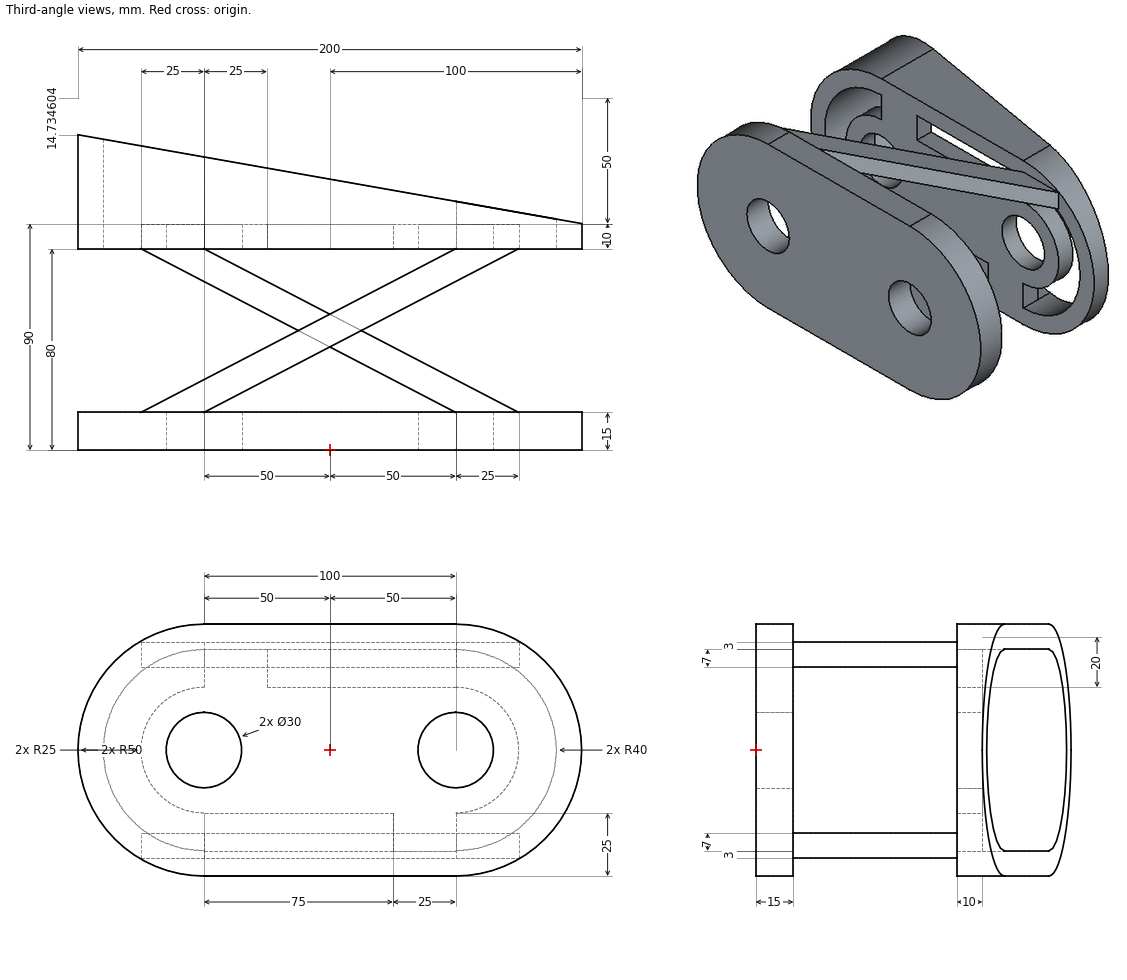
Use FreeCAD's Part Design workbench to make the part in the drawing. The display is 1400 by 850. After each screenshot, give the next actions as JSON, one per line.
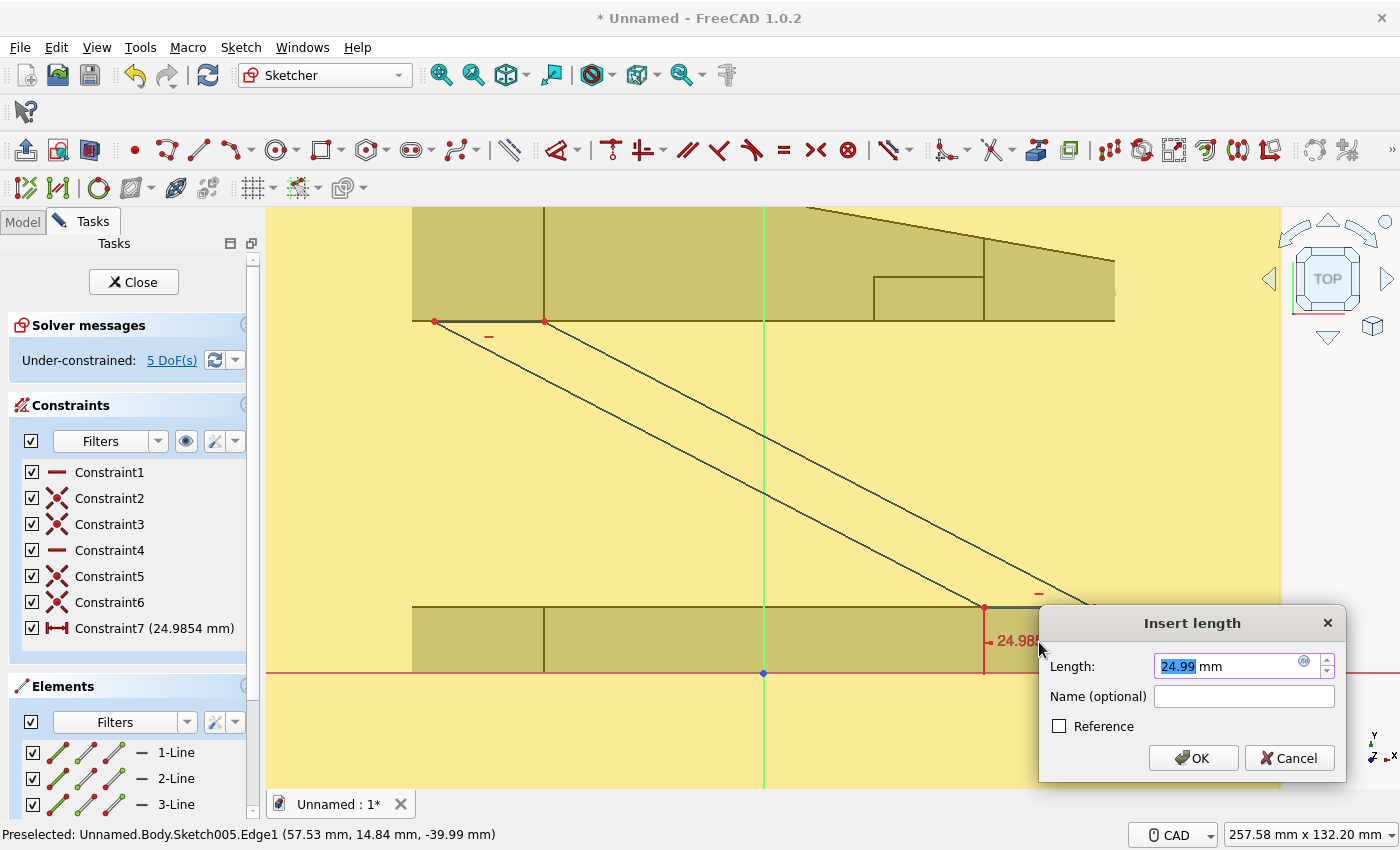
{"action": "type", "text": "25"}
{"action": "key", "text": "Return"}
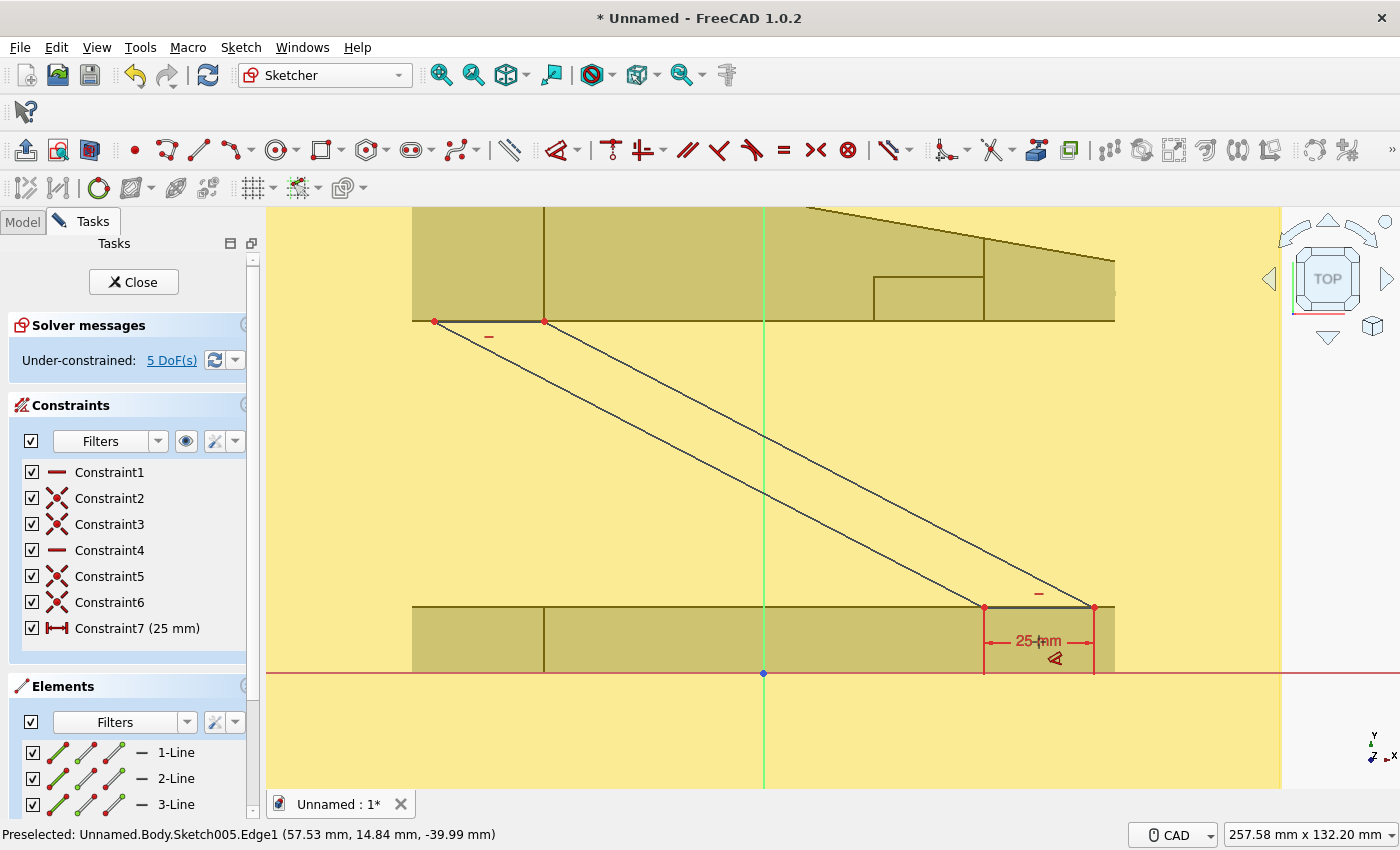
{"action": "left_click", "coordinate": [511, 322]}
{"action": "left_click", "coordinate": [489, 288]}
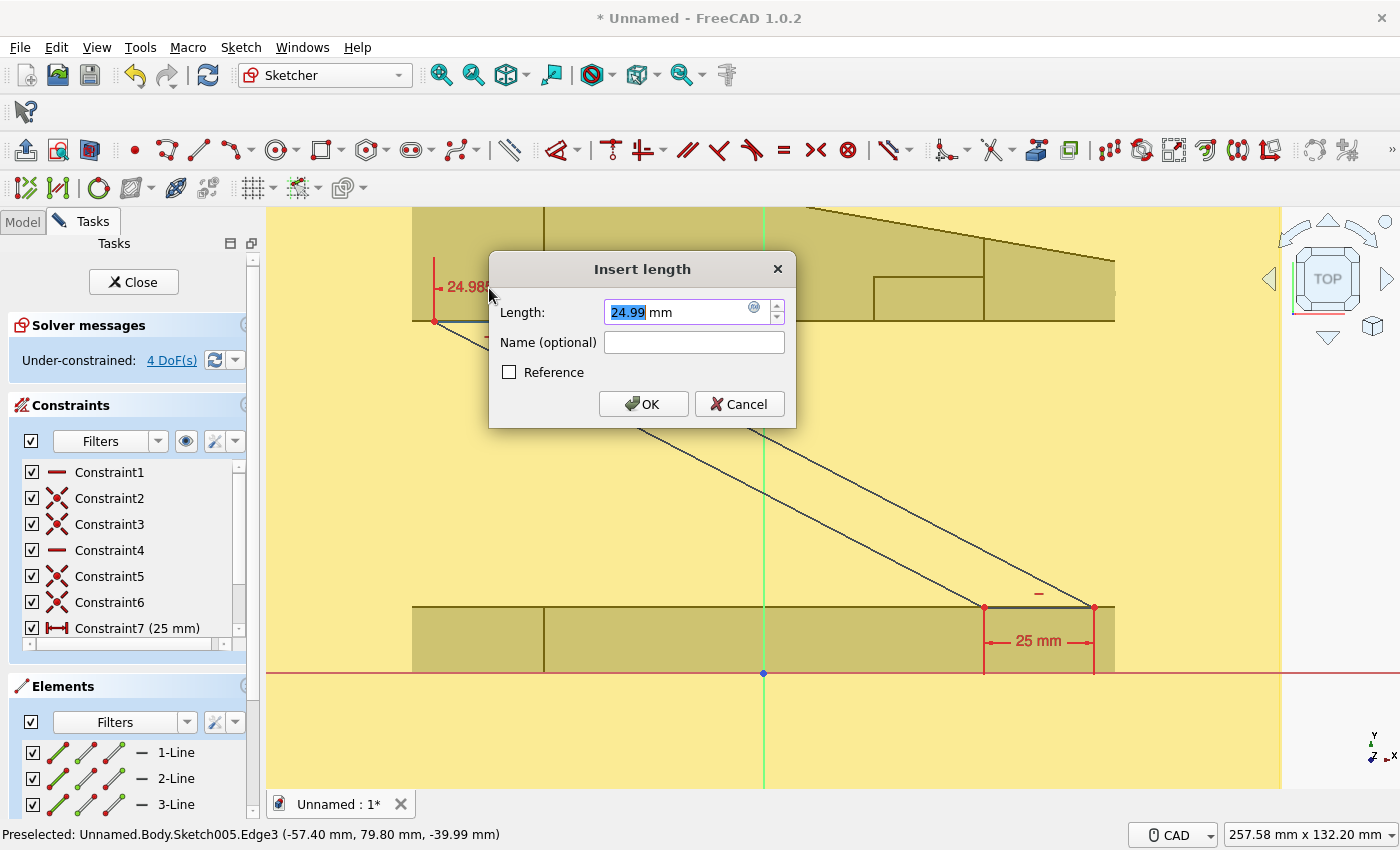
{"action": "type", "text": "25"}
{"action": "key", "text": "Return"}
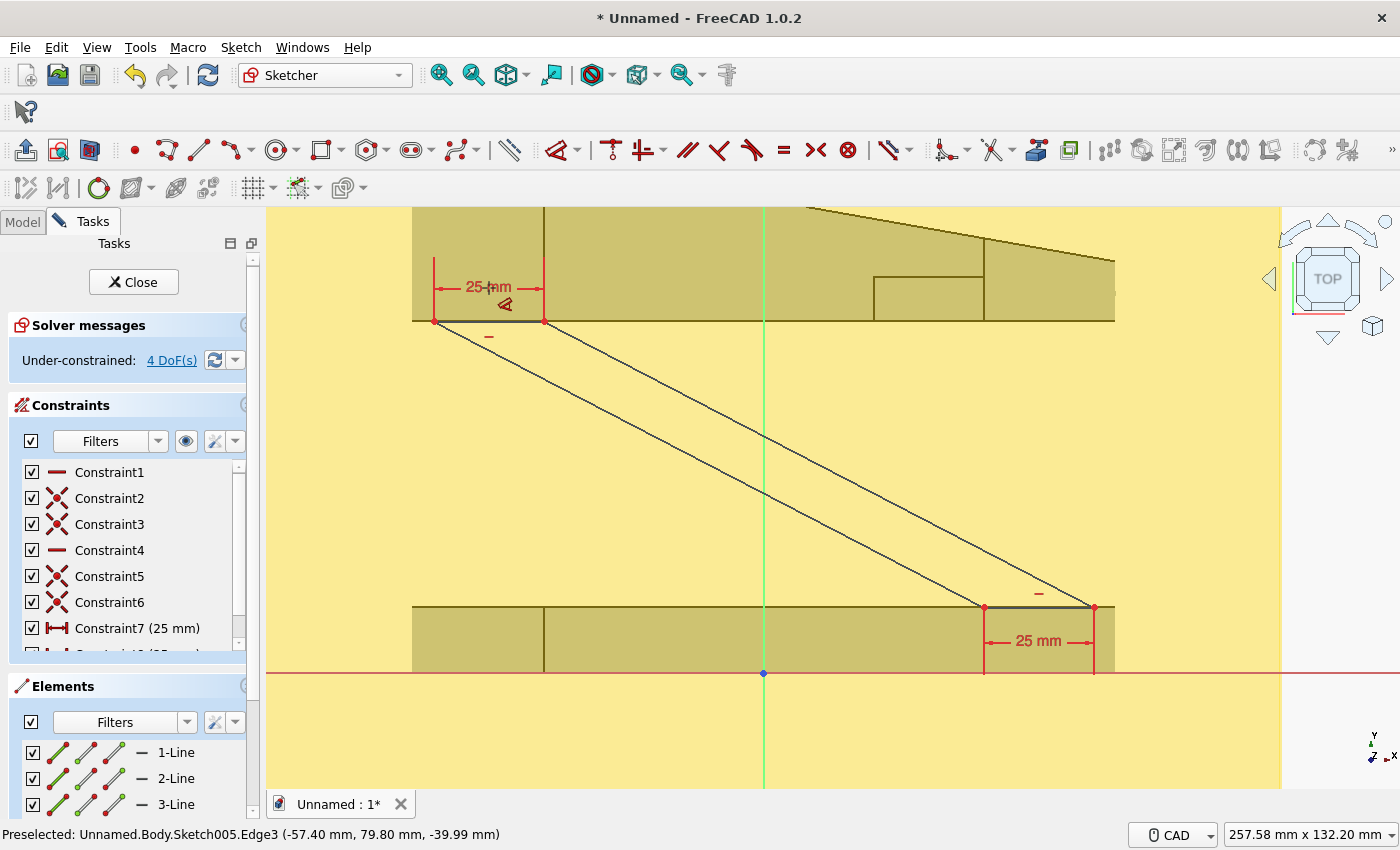
{"action": "left_click", "coordinate": [984, 608]}
{"action": "left_click", "coordinate": [874, 707]}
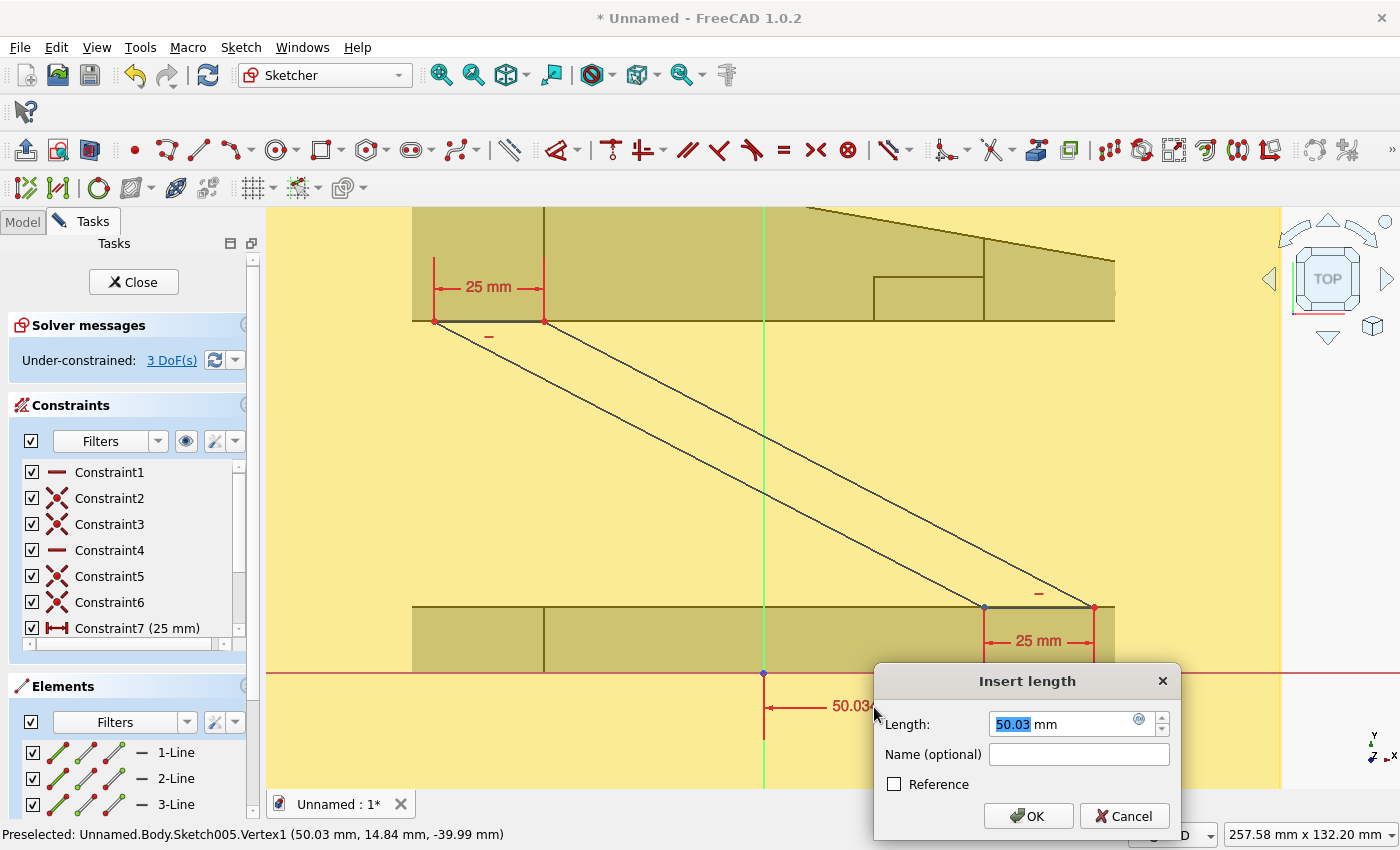
{"action": "type", "text": "50"}
{"action": "key", "text": "Return"}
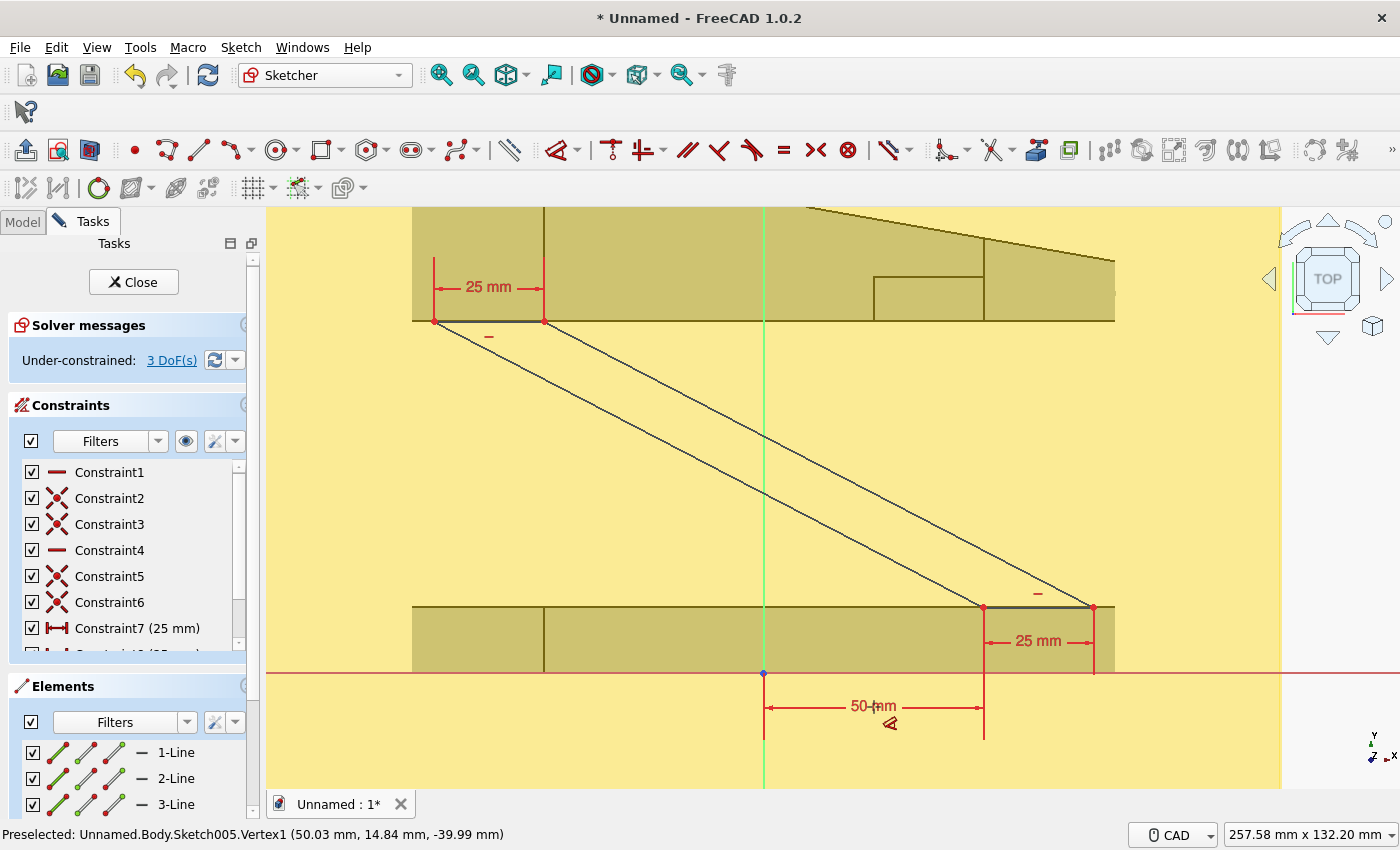
{"action": "left_click", "coordinate": [984, 608]}
{"action": "left_click", "coordinate": [730, 641]}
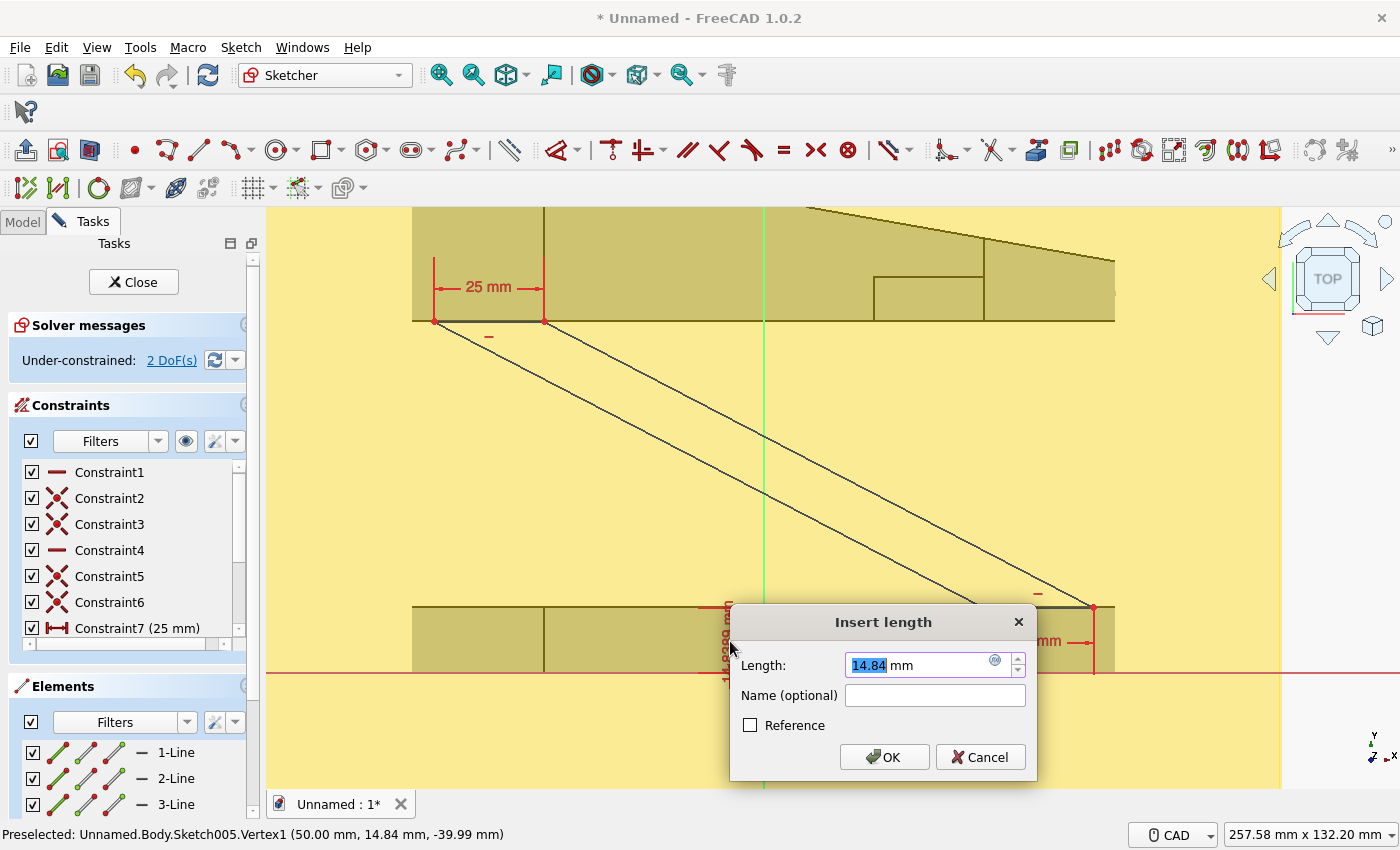
{"action": "type", "text": "15"}
{"action": "key", "text": "Return"}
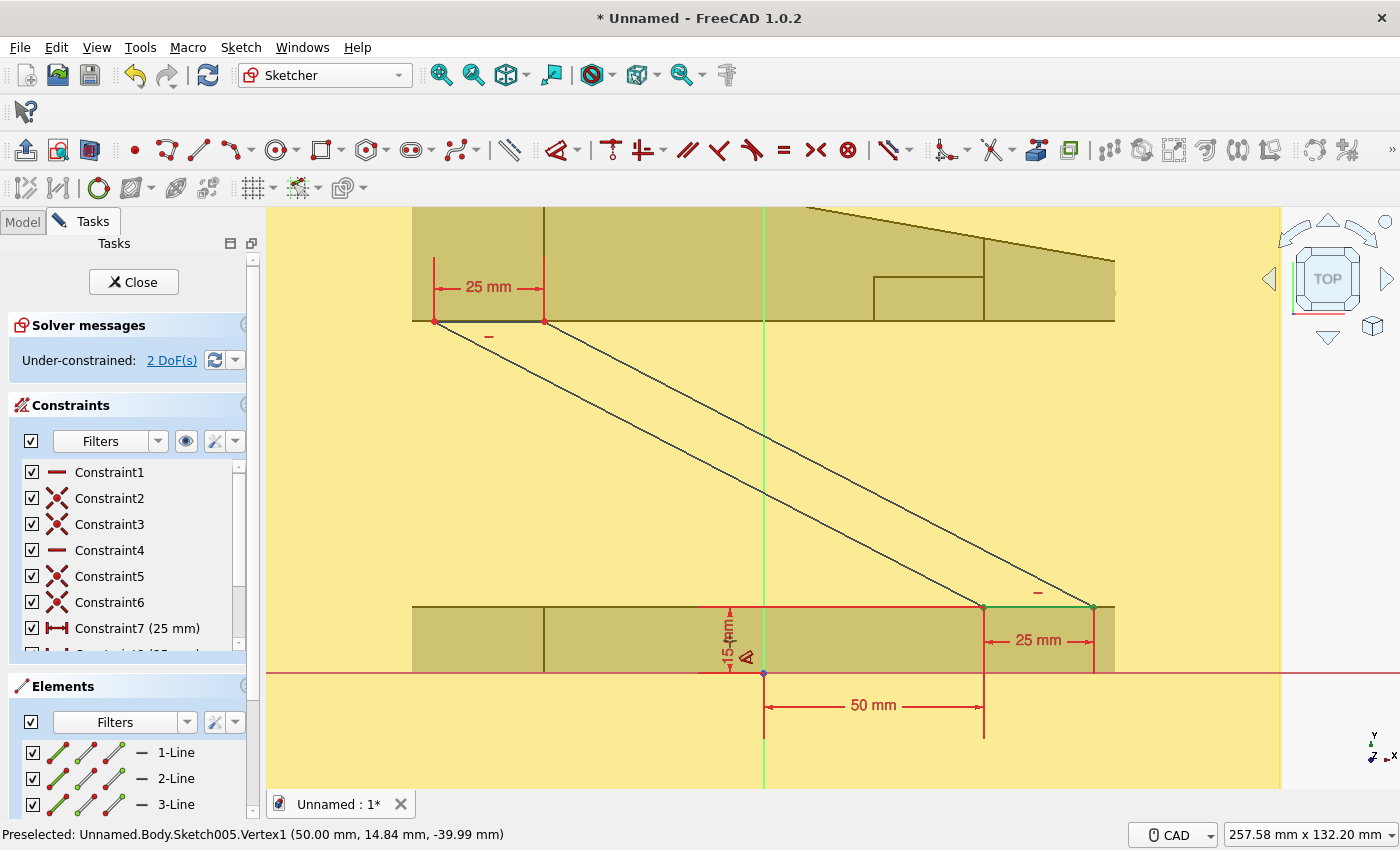
{"action": "left_click", "coordinate": [544, 322]}
{"action": "left_click", "coordinate": [654, 707]}